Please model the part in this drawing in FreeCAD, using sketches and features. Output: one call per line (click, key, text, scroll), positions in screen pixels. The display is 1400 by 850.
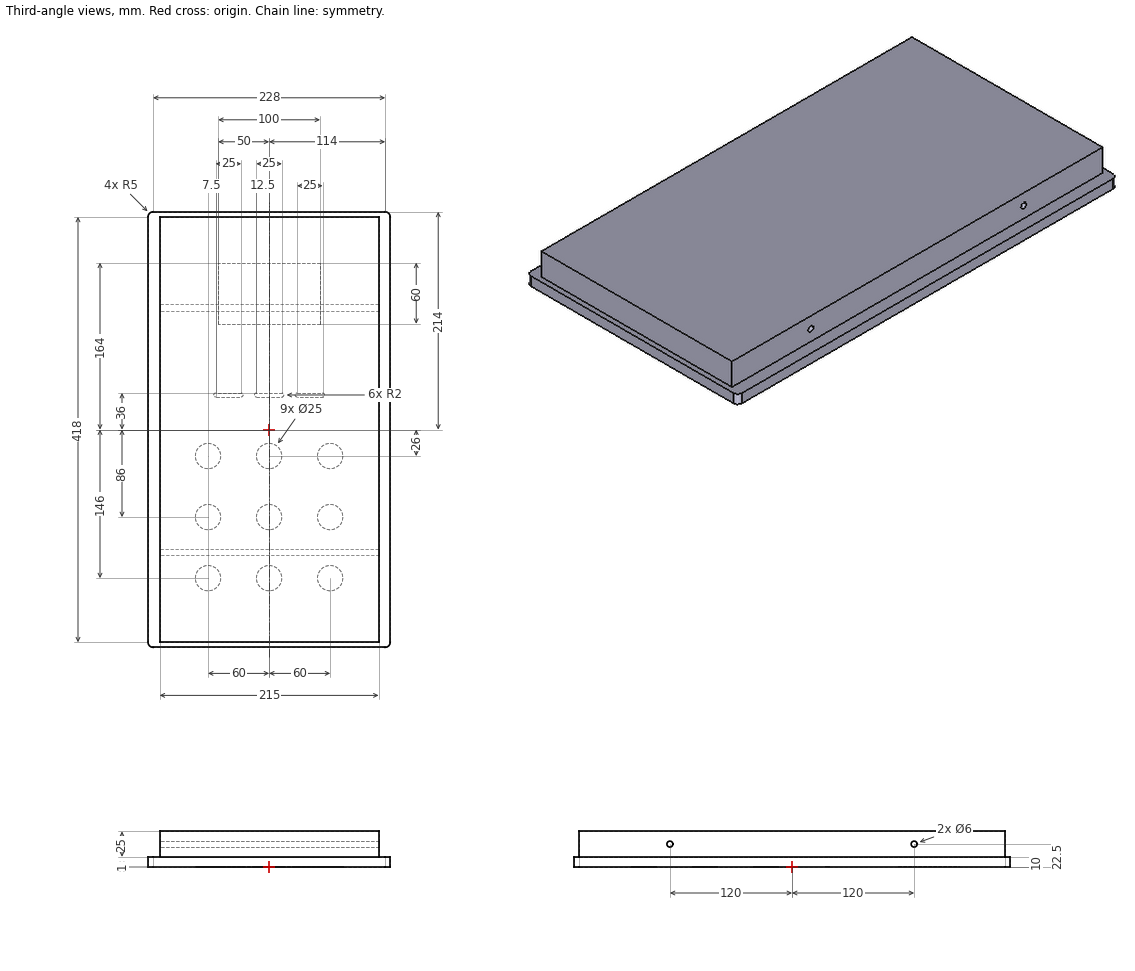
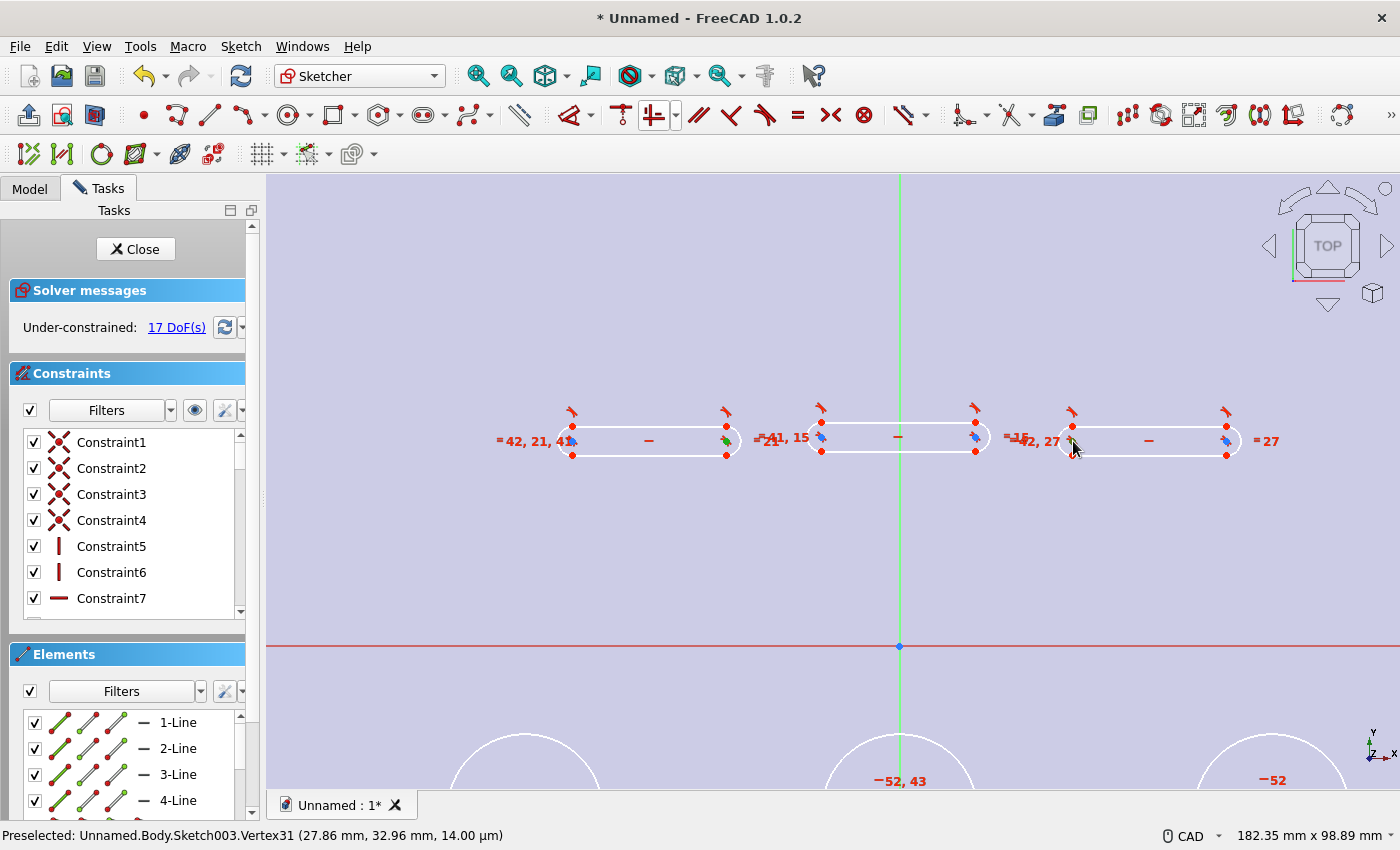
click(900, 681)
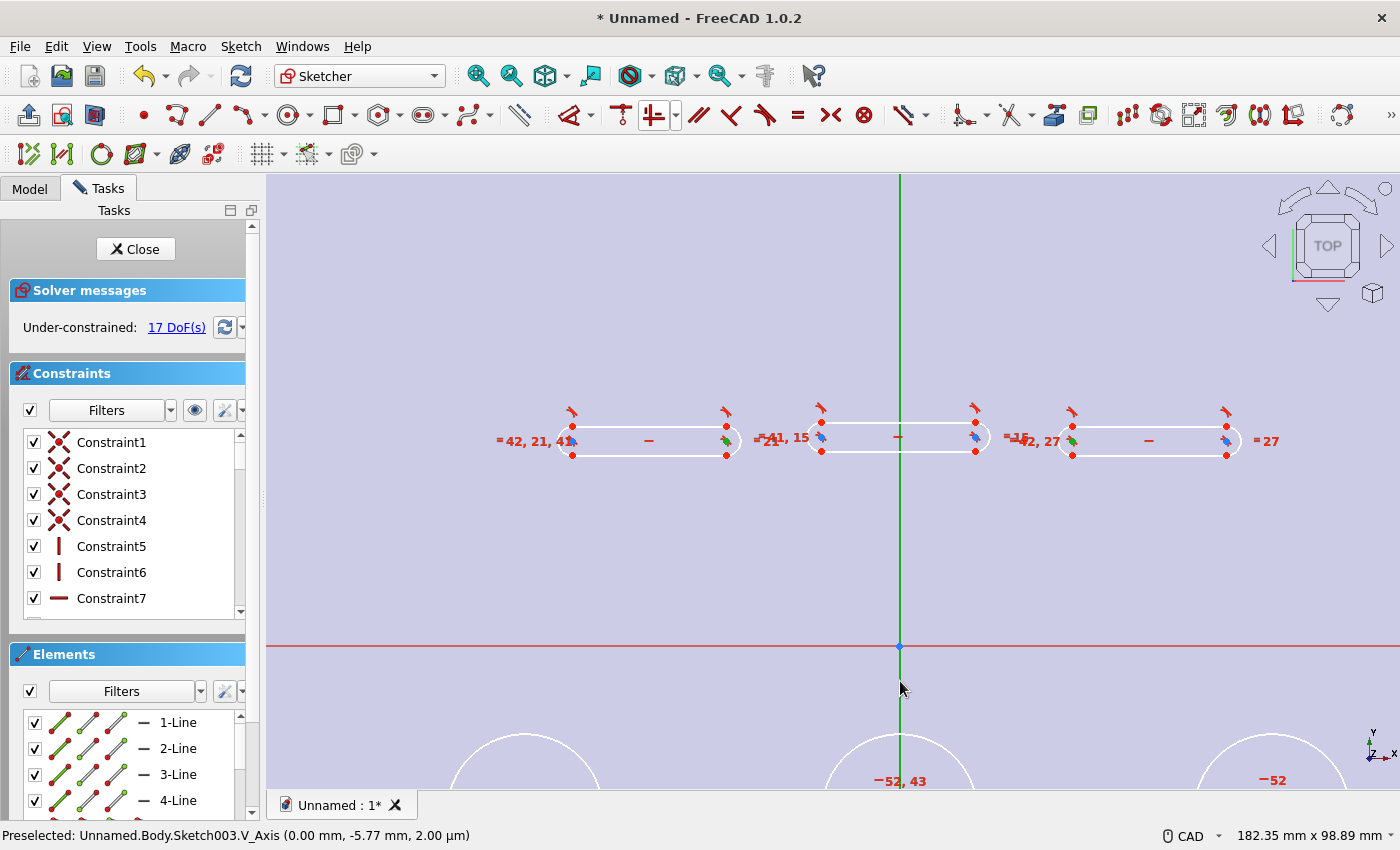
key(s)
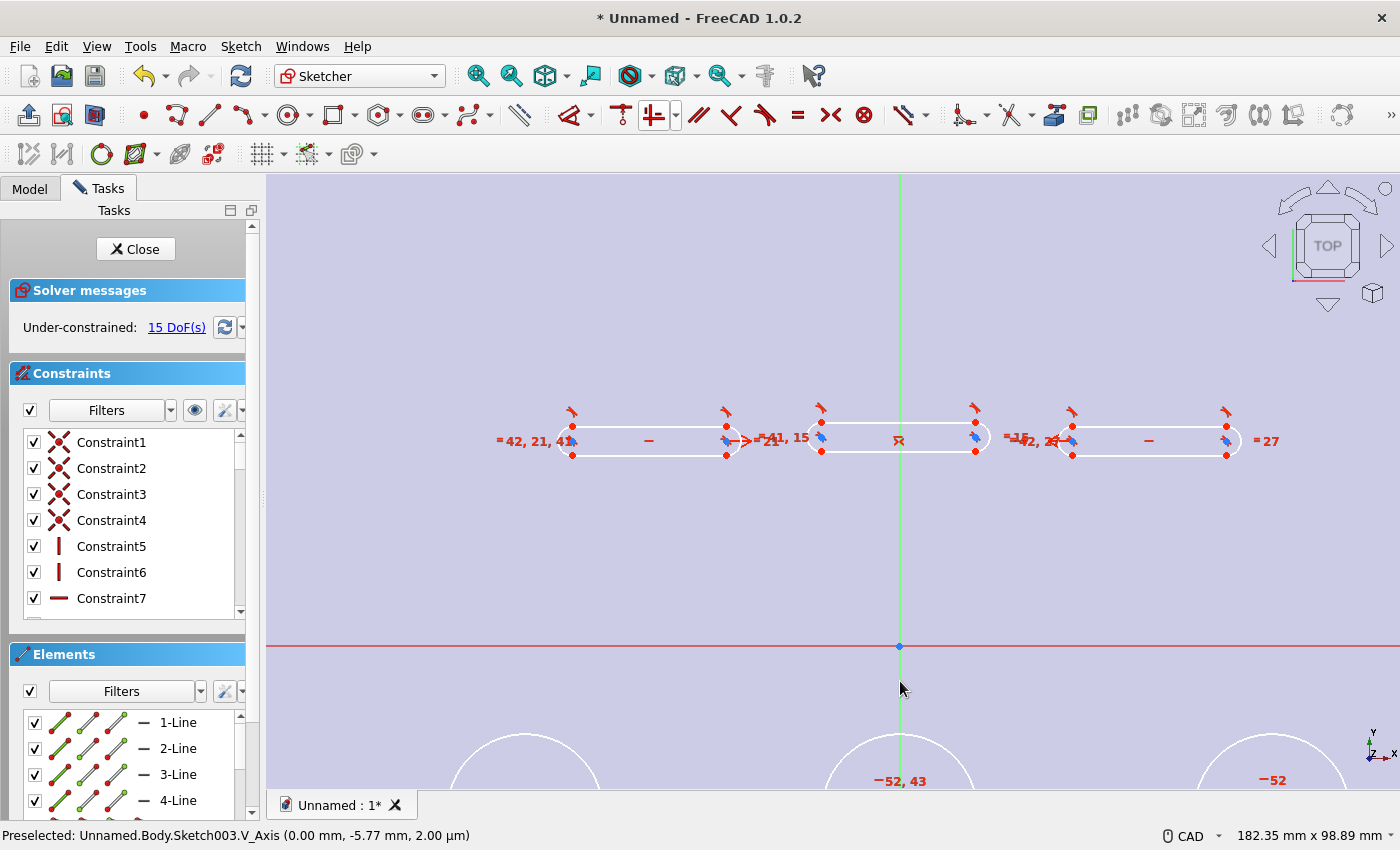
click(568, 116)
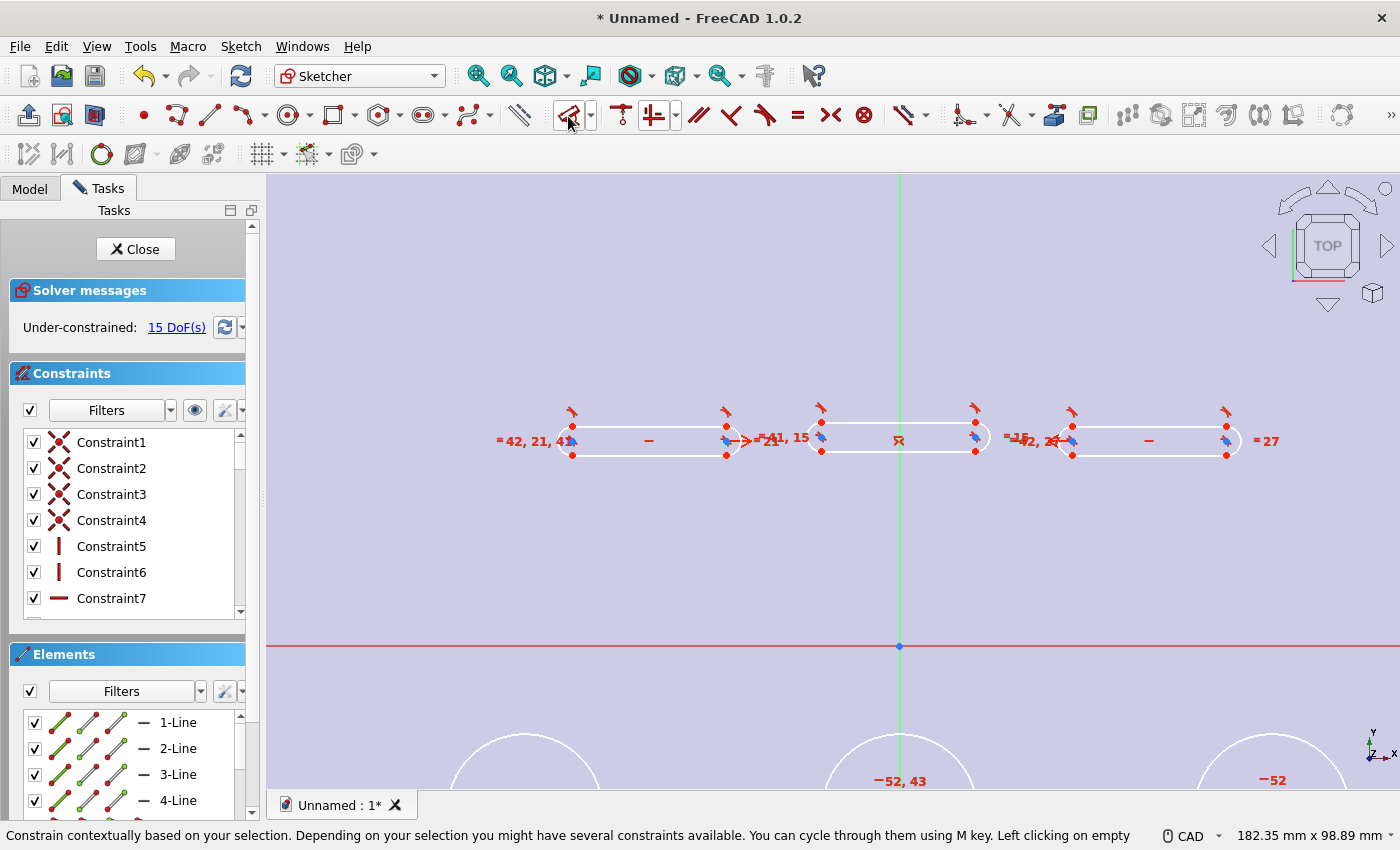
scroll(810, 429, up, 6)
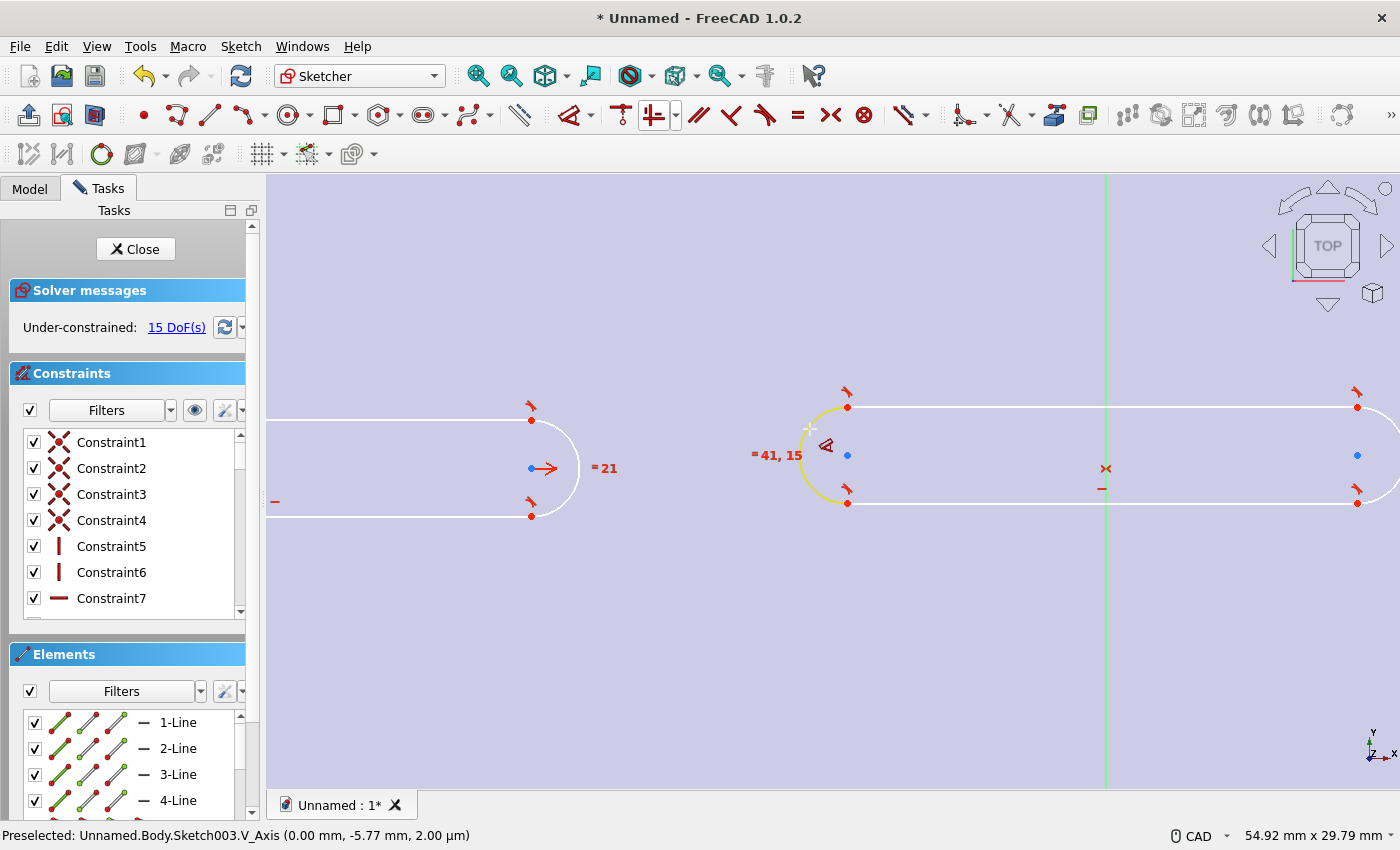
click(809, 427)
click(783, 408)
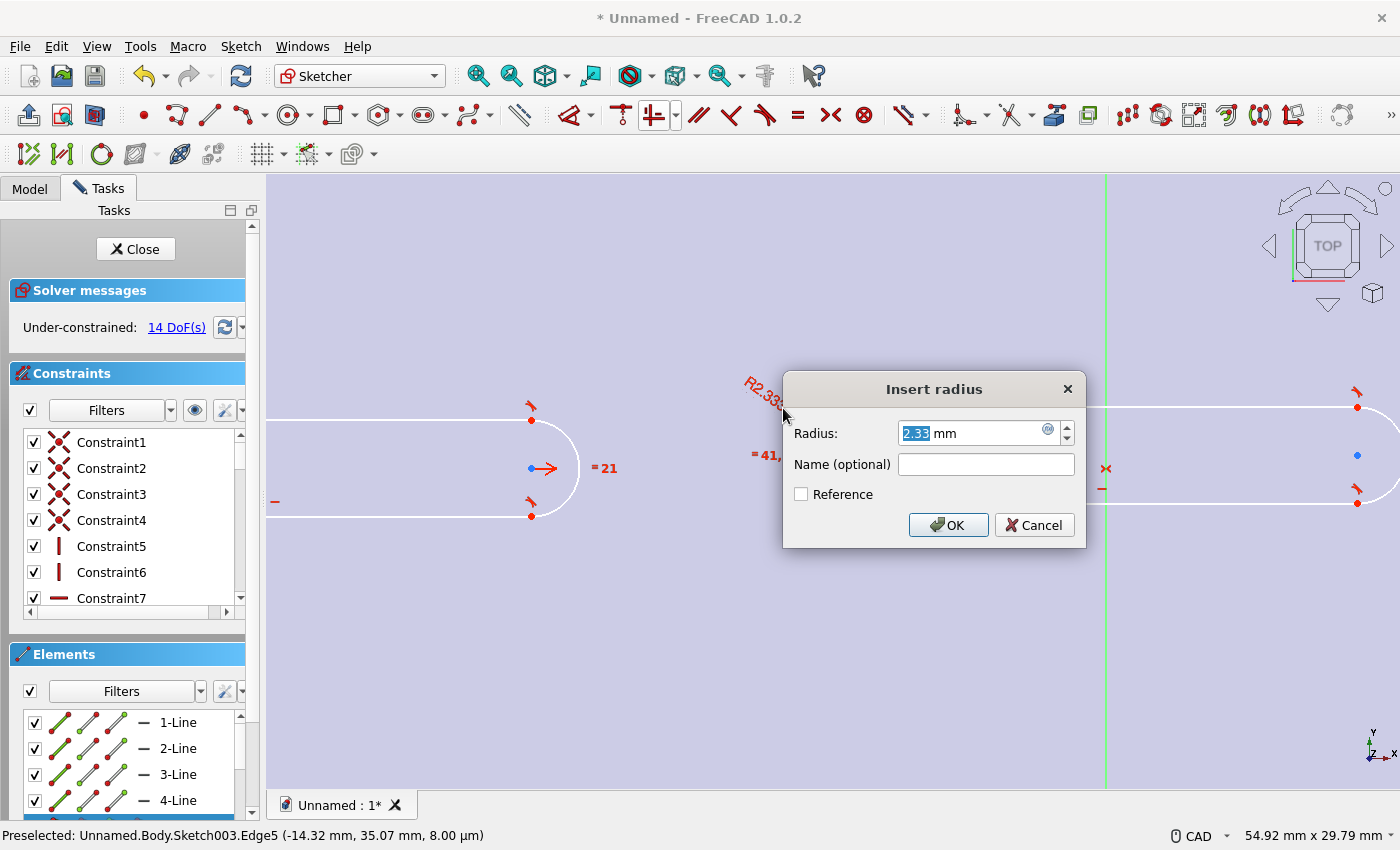
text(2)
key(Return)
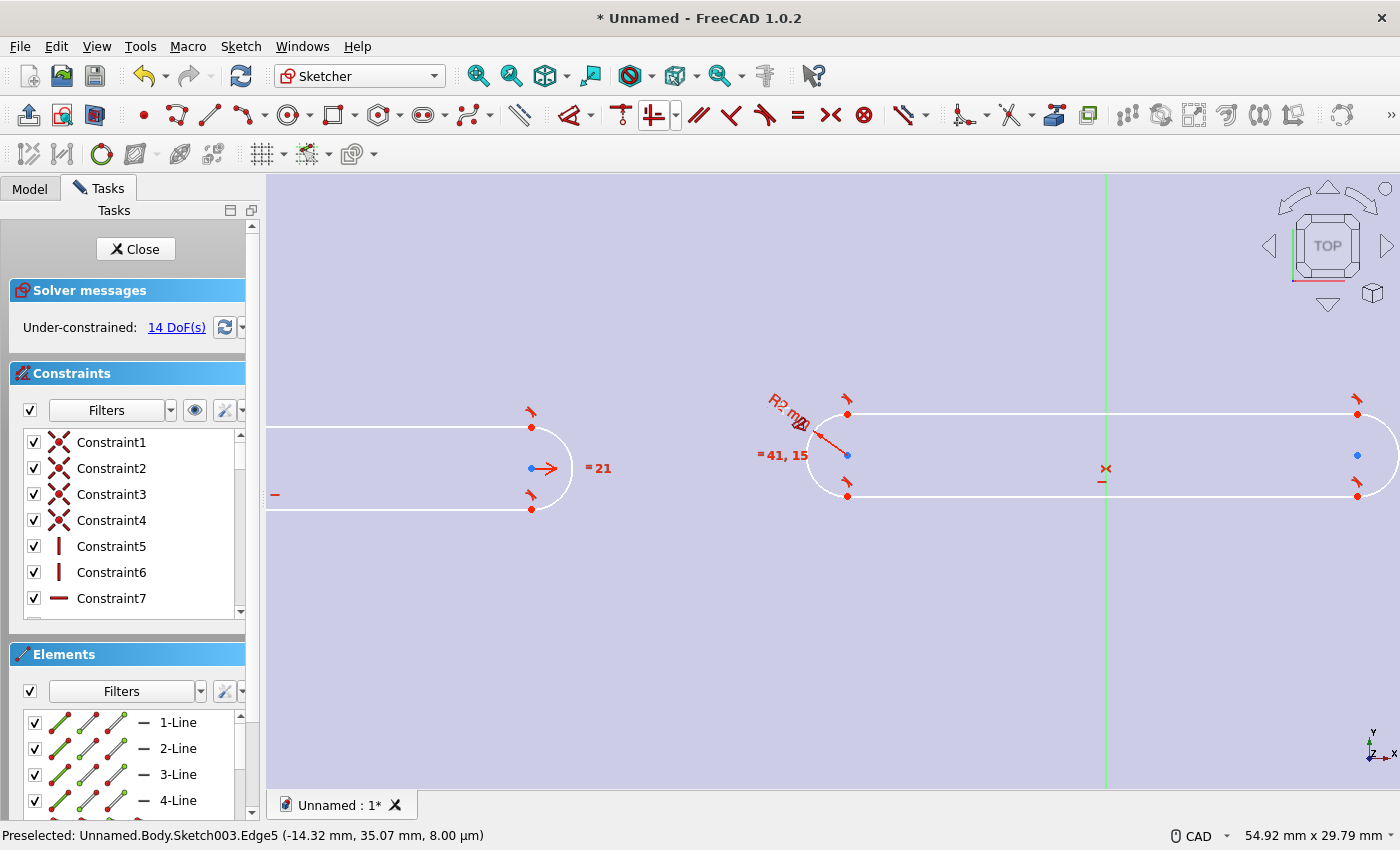
scroll(742, 442, down, 14)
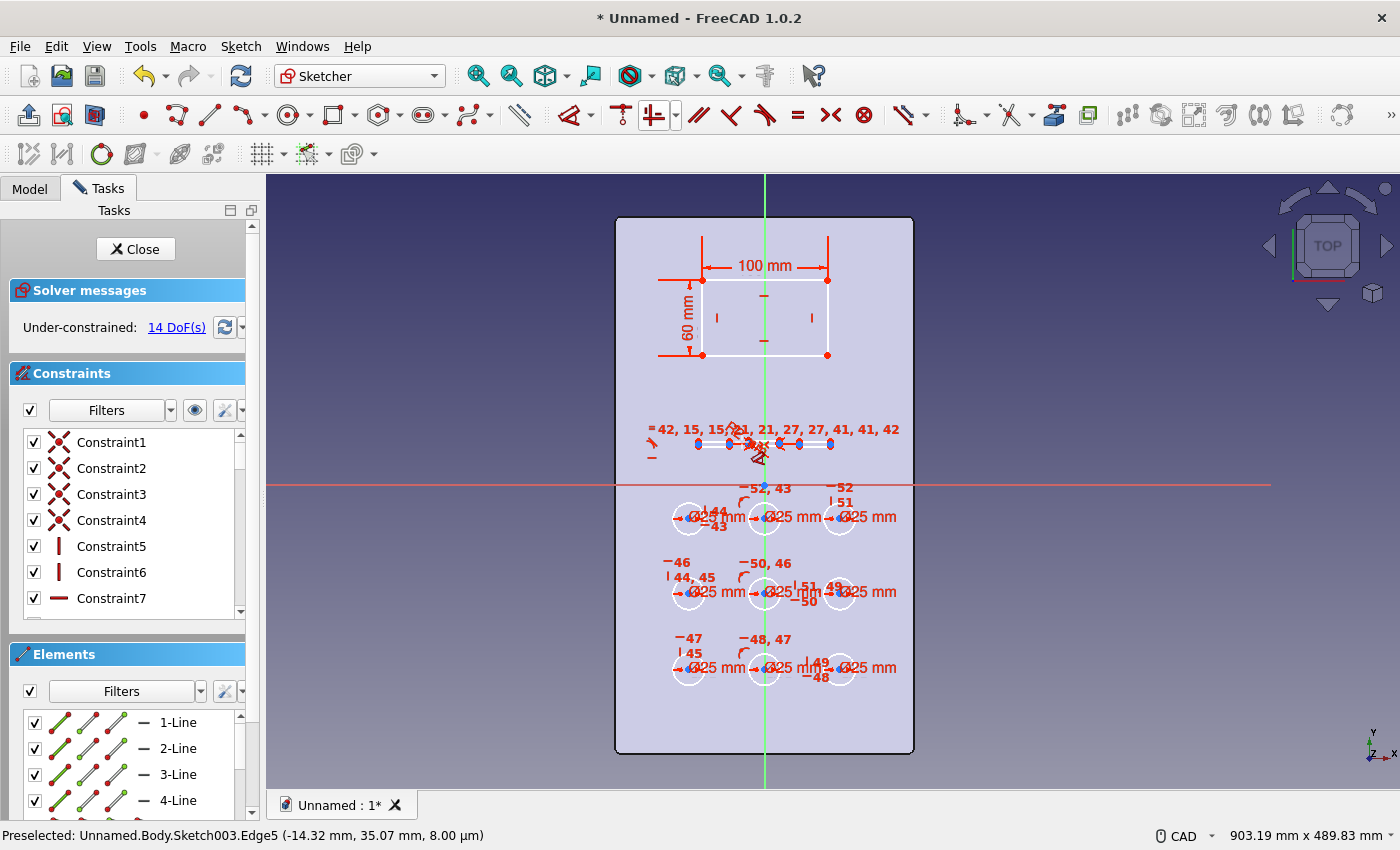
scroll(758, 441, up, 6)